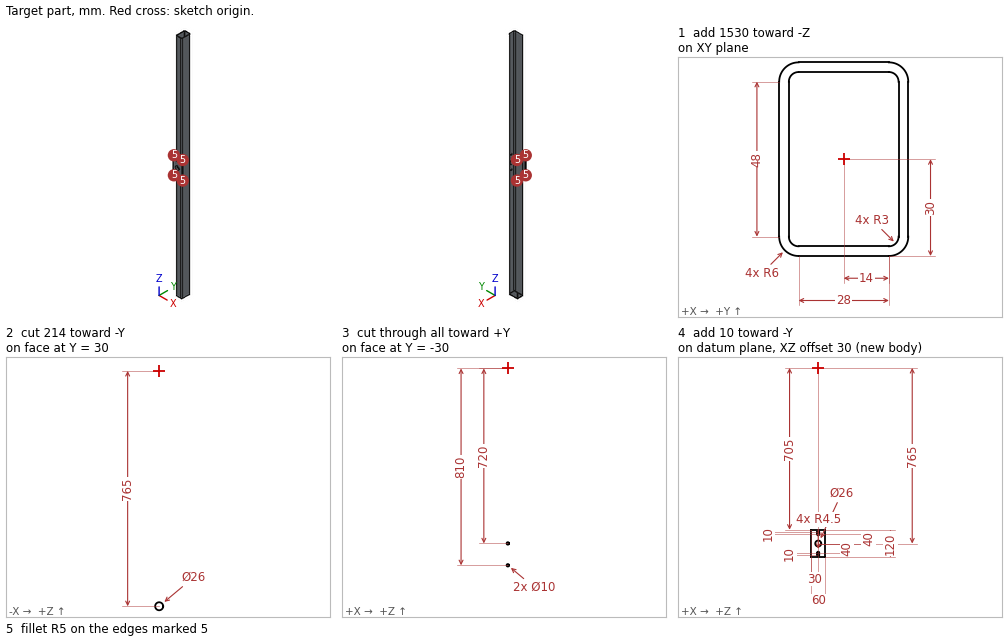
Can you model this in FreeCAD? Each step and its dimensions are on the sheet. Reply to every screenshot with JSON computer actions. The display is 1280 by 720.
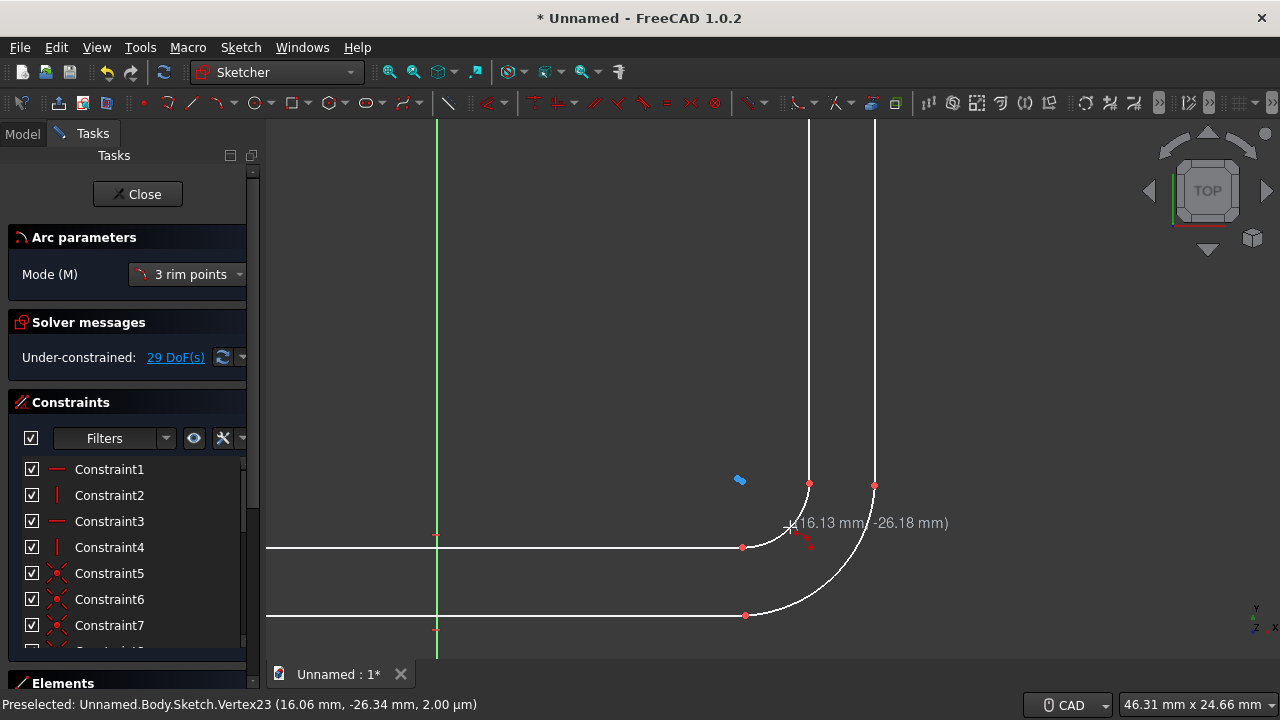
{"action": "scroll", "coordinate": [792, 531], "scroll_direction": "down", "scroll_amount": 7}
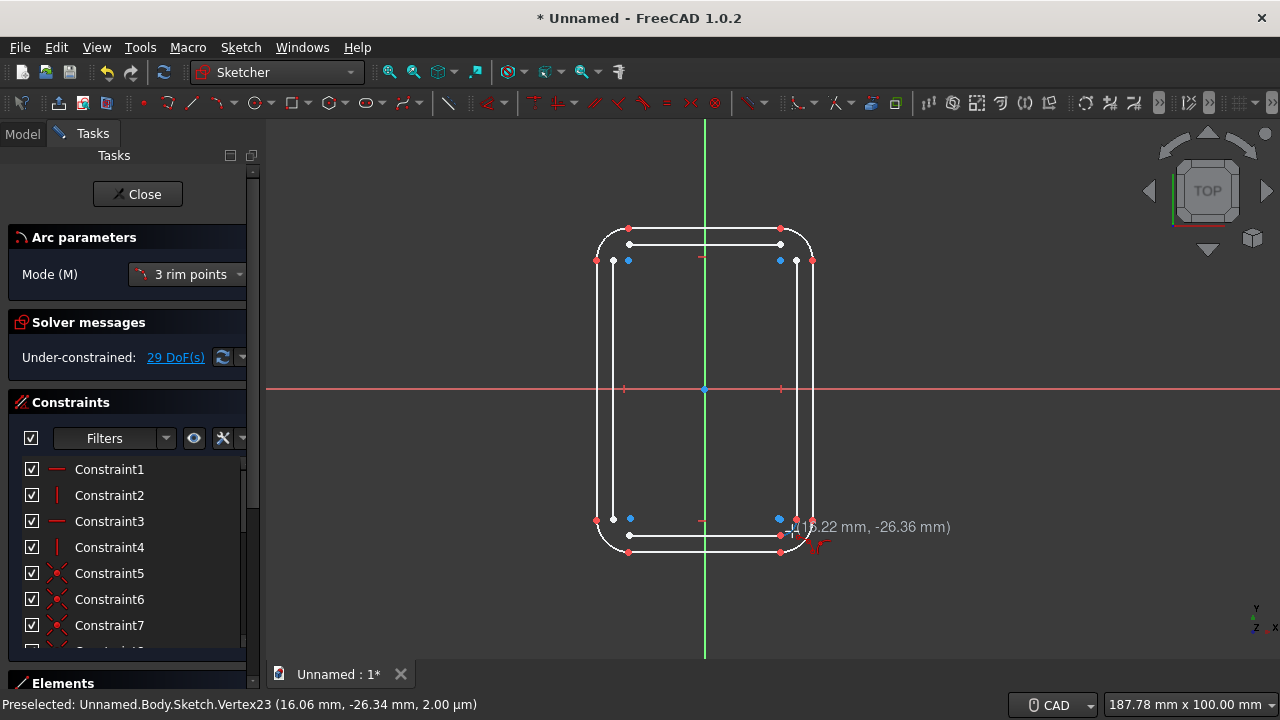
{"action": "left_click", "coordinate": [797, 261]}
{"action": "left_click", "coordinate": [780, 245]}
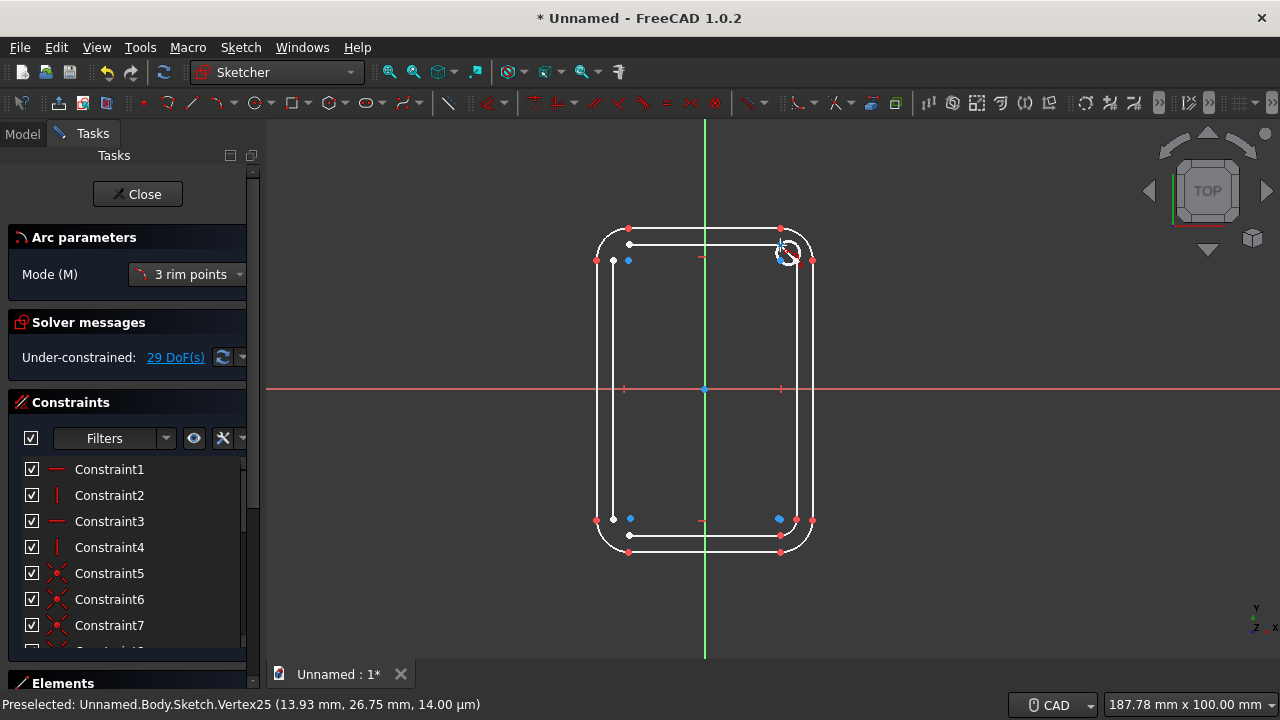
{"action": "scroll", "coordinate": [792, 248], "scroll_direction": "up", "scroll_amount": 7}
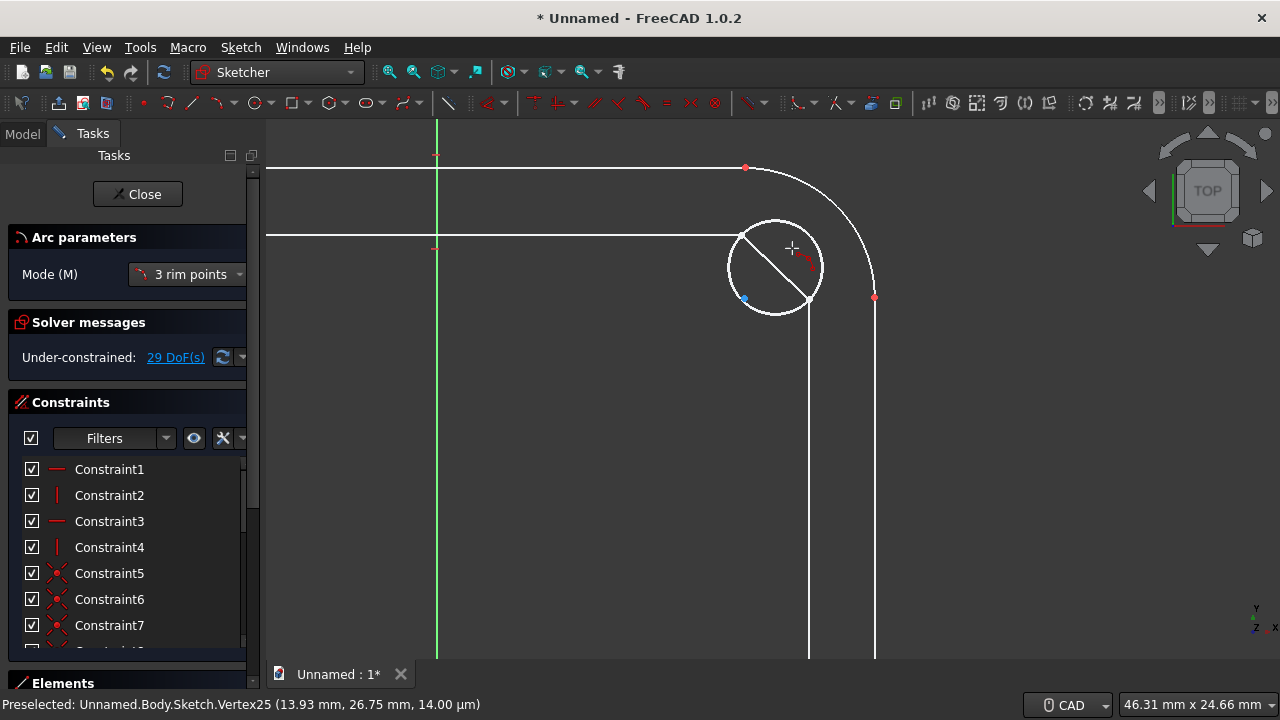
{"action": "left_click", "coordinate": [790, 249]}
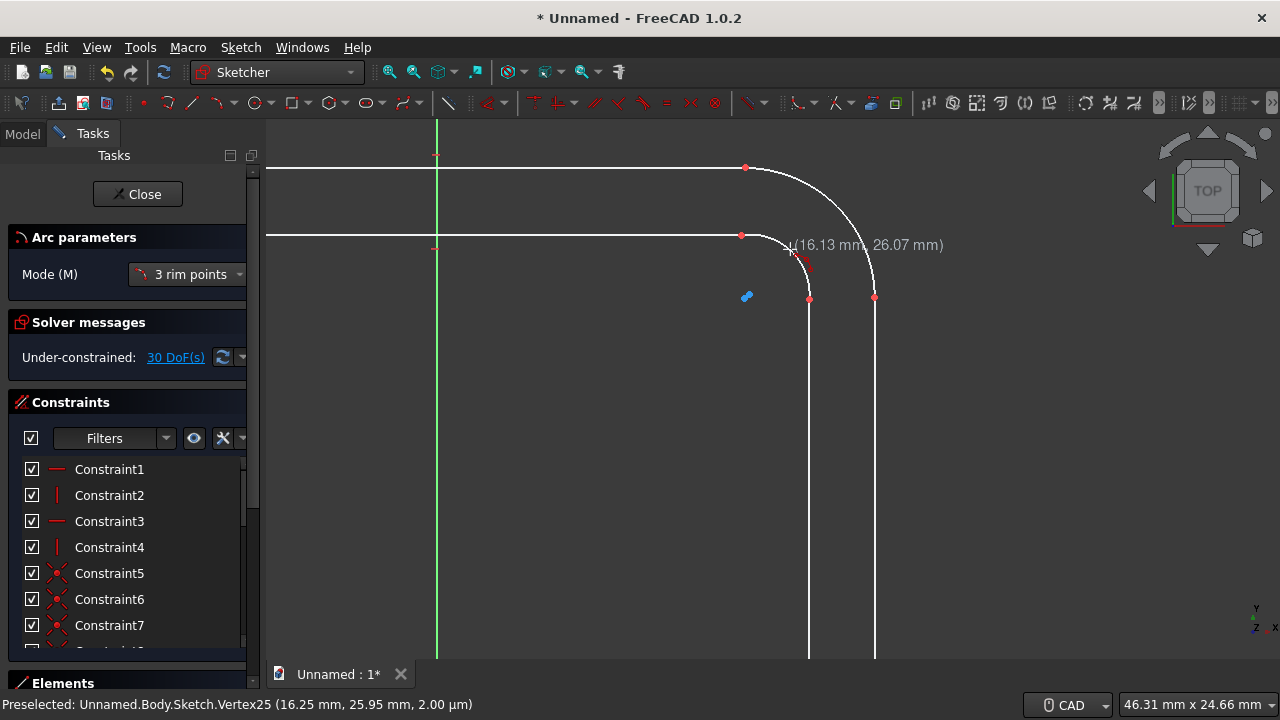
{"action": "scroll", "coordinate": [792, 248], "scroll_direction": "down", "scroll_amount": 7}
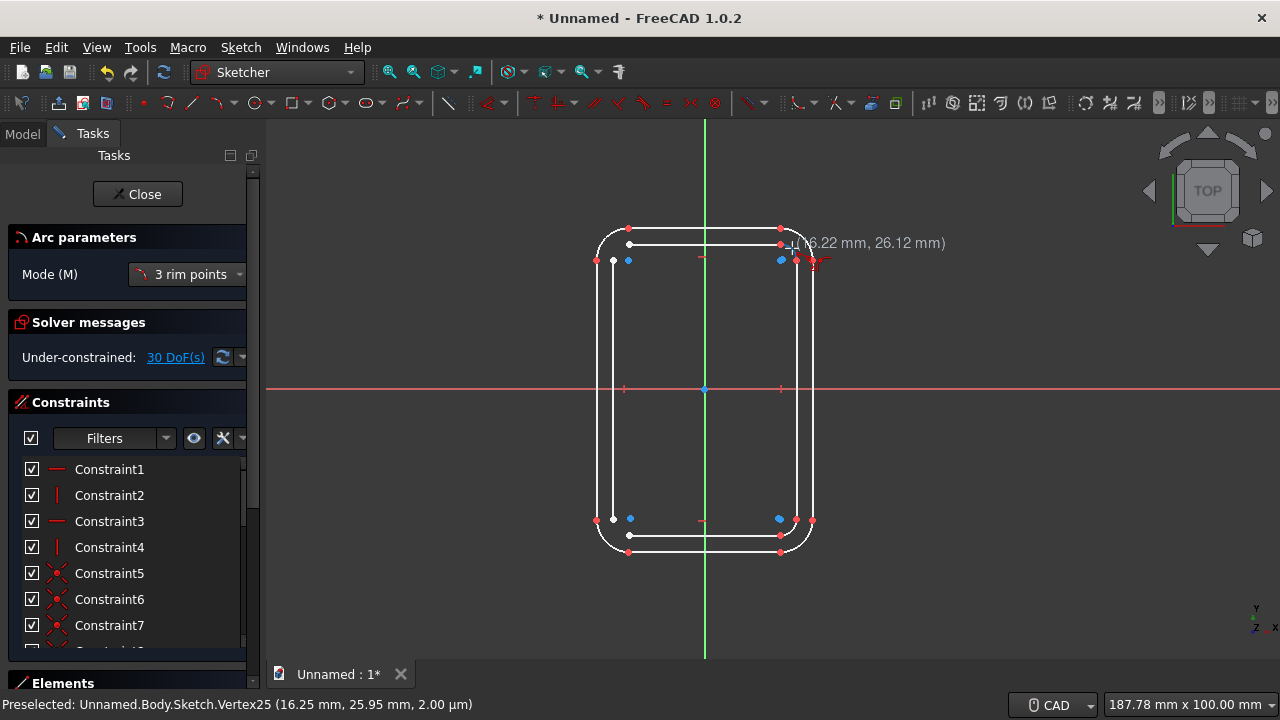
{"action": "left_click", "coordinate": [629, 245]}
{"action": "left_click", "coordinate": [613, 261]}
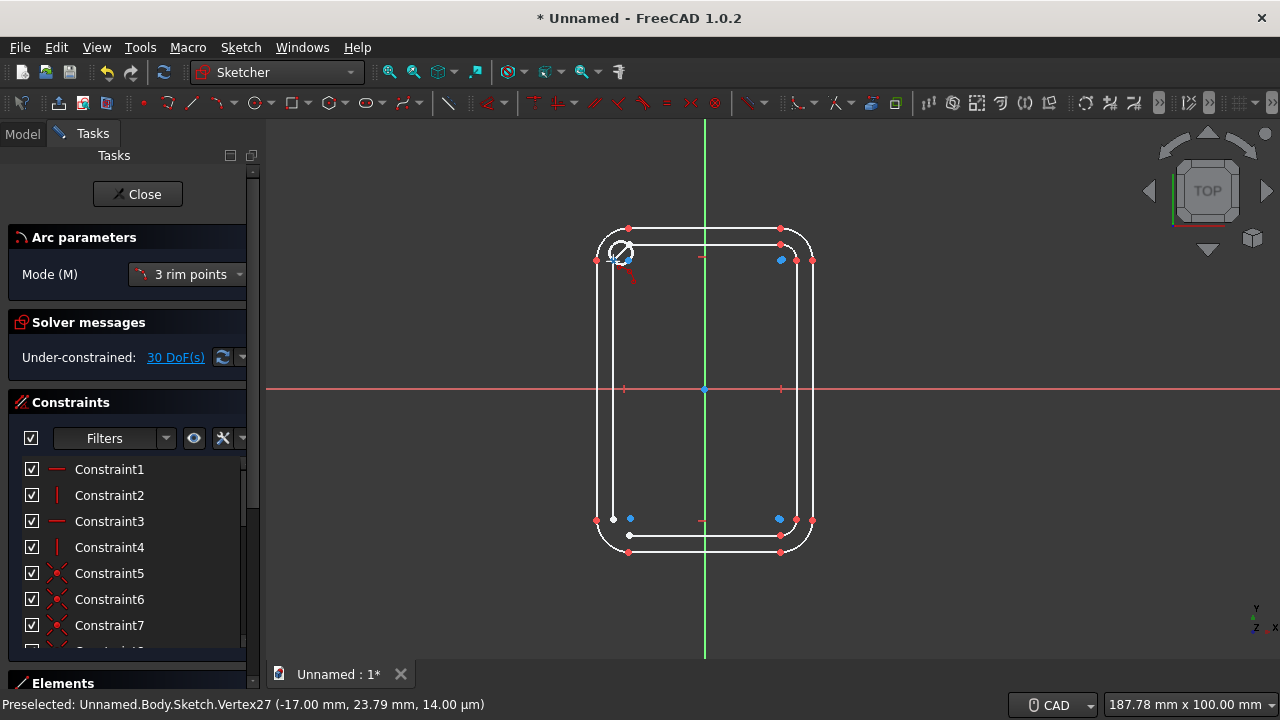
{"action": "scroll", "coordinate": [618, 248], "scroll_direction": "up", "scroll_amount": 7}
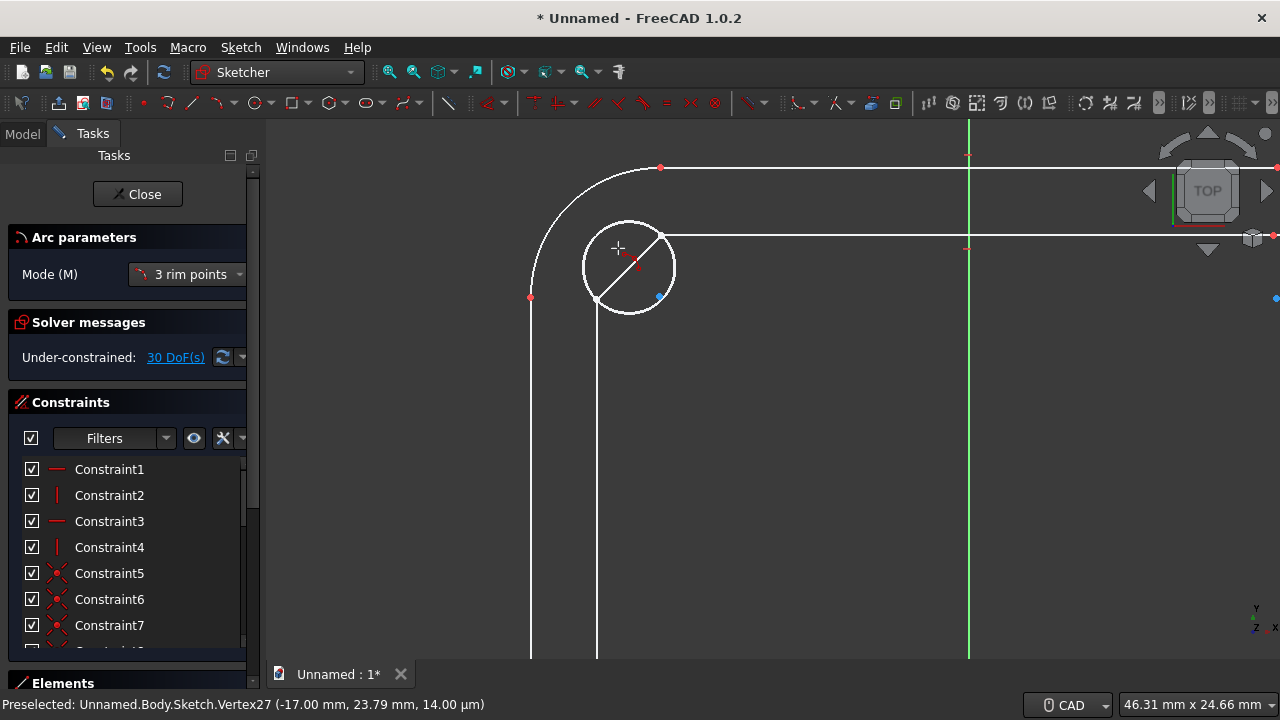
{"action": "left_click", "coordinate": [616, 249]}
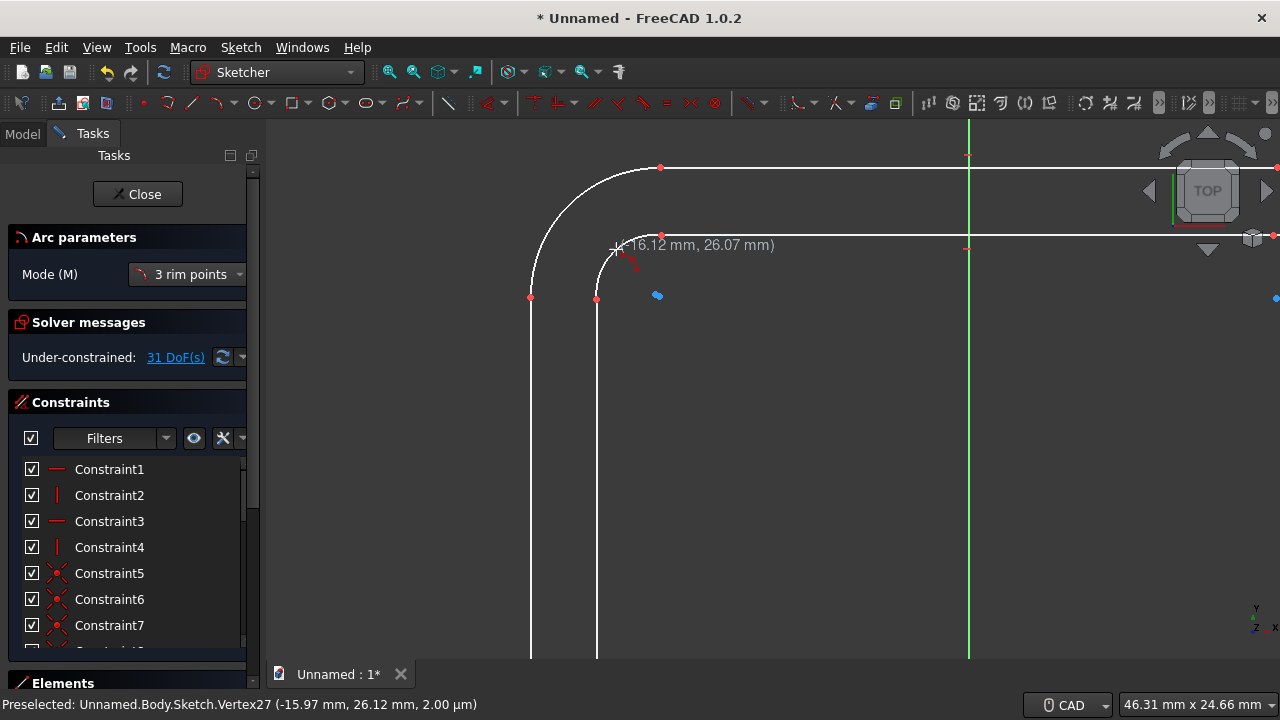
{"action": "scroll", "coordinate": [618, 248], "scroll_direction": "down", "scroll_amount": 7}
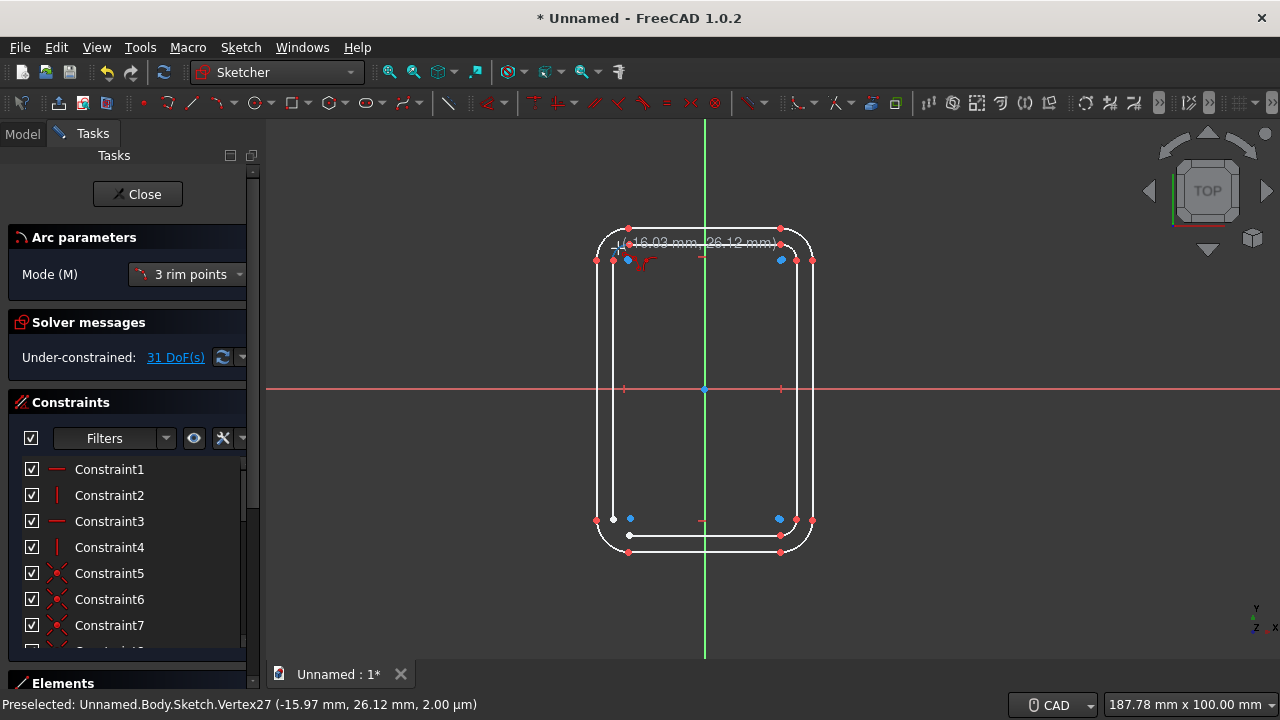
{"action": "left_click", "coordinate": [613, 520]}
{"action": "left_click", "coordinate": [629, 536]}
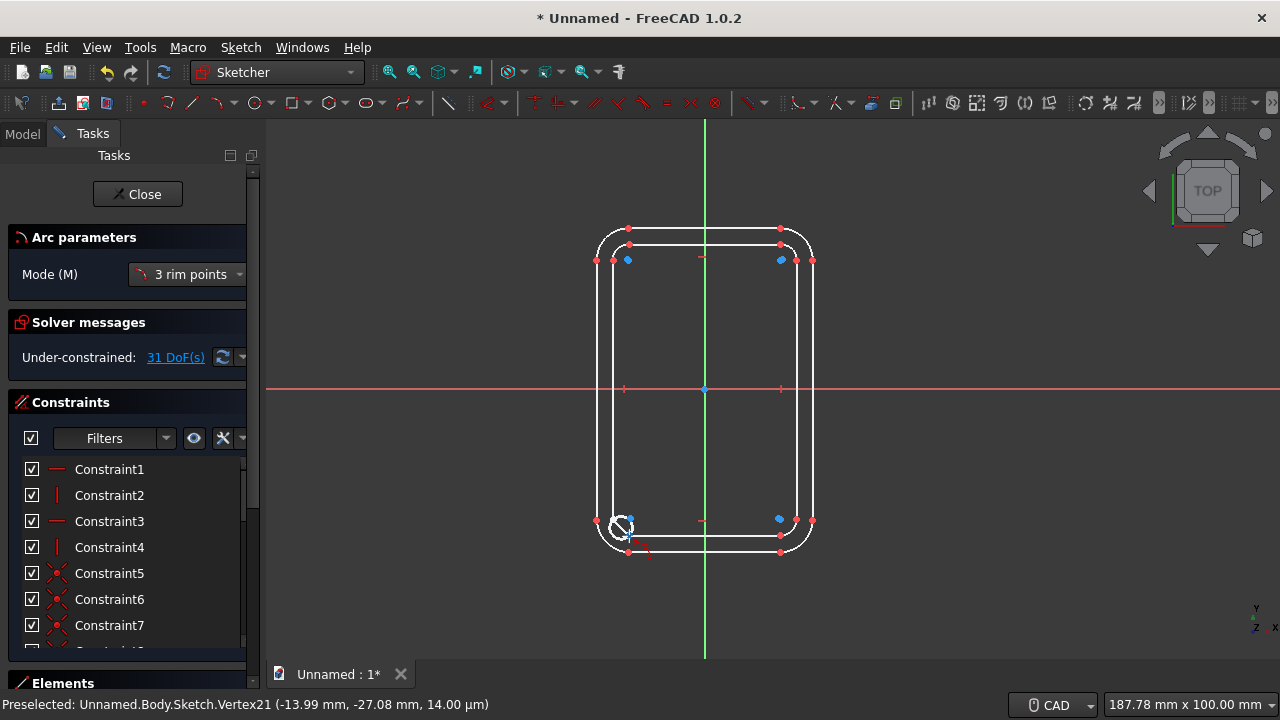
{"action": "scroll", "coordinate": [618, 531], "scroll_direction": "up", "scroll_amount": 7}